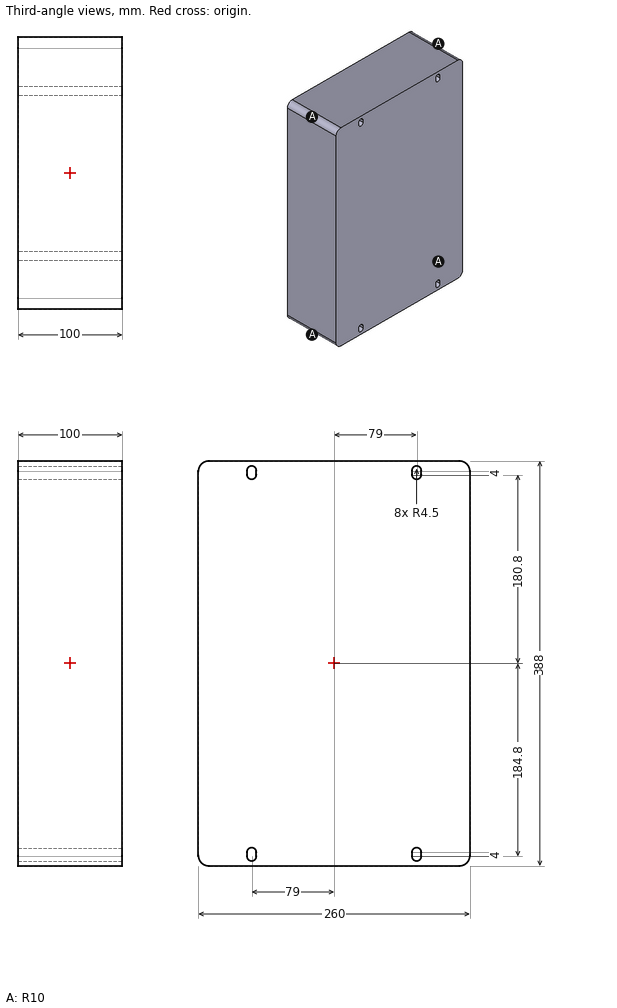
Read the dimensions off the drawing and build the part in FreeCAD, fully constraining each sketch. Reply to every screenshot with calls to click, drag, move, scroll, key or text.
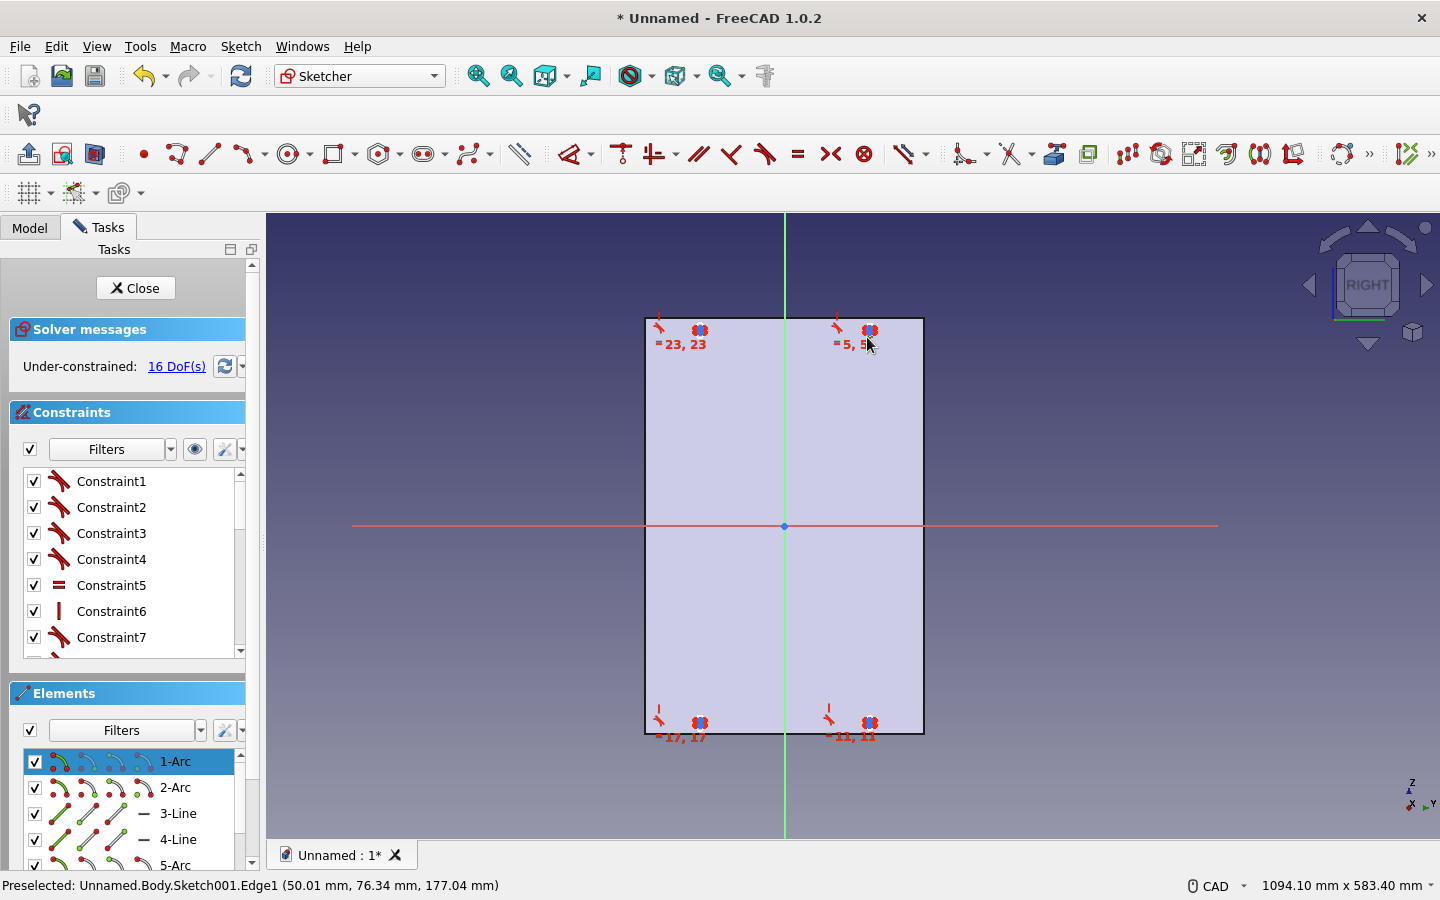
scroll(867, 729, up, 6)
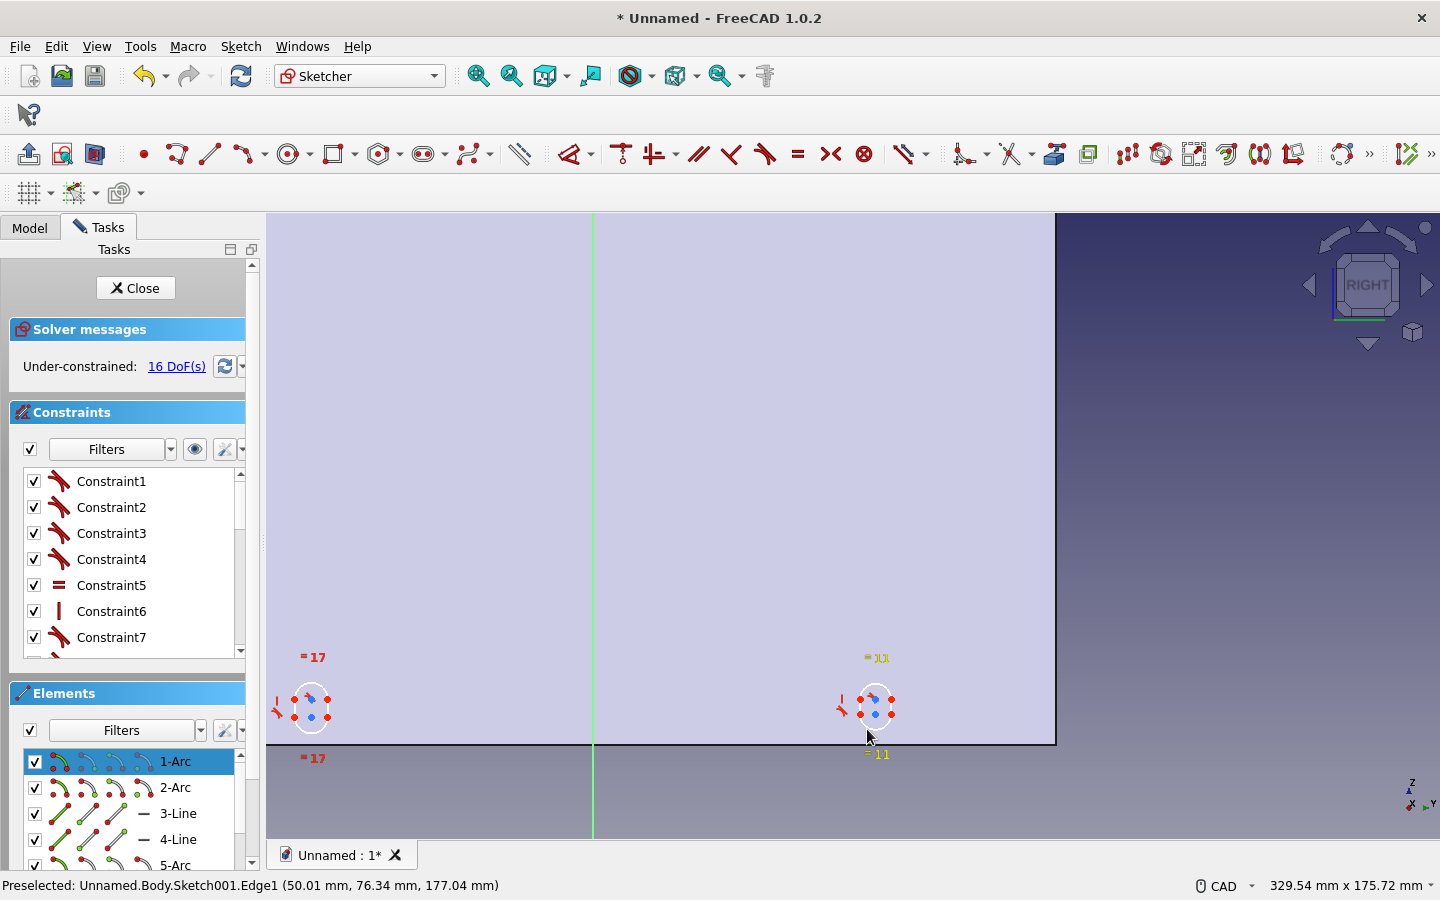
click(866, 727)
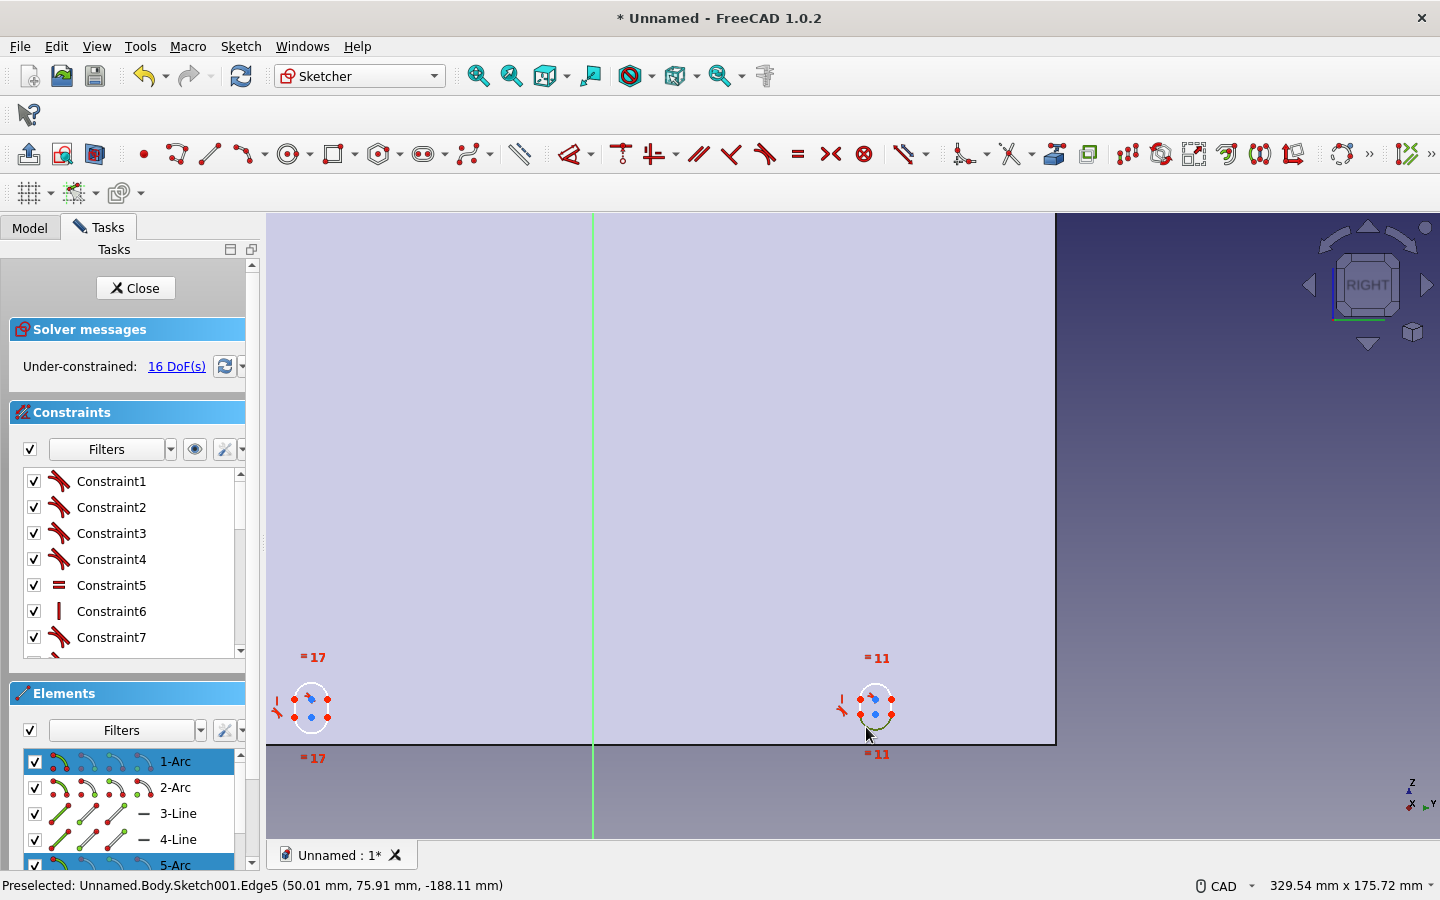
click(302, 730)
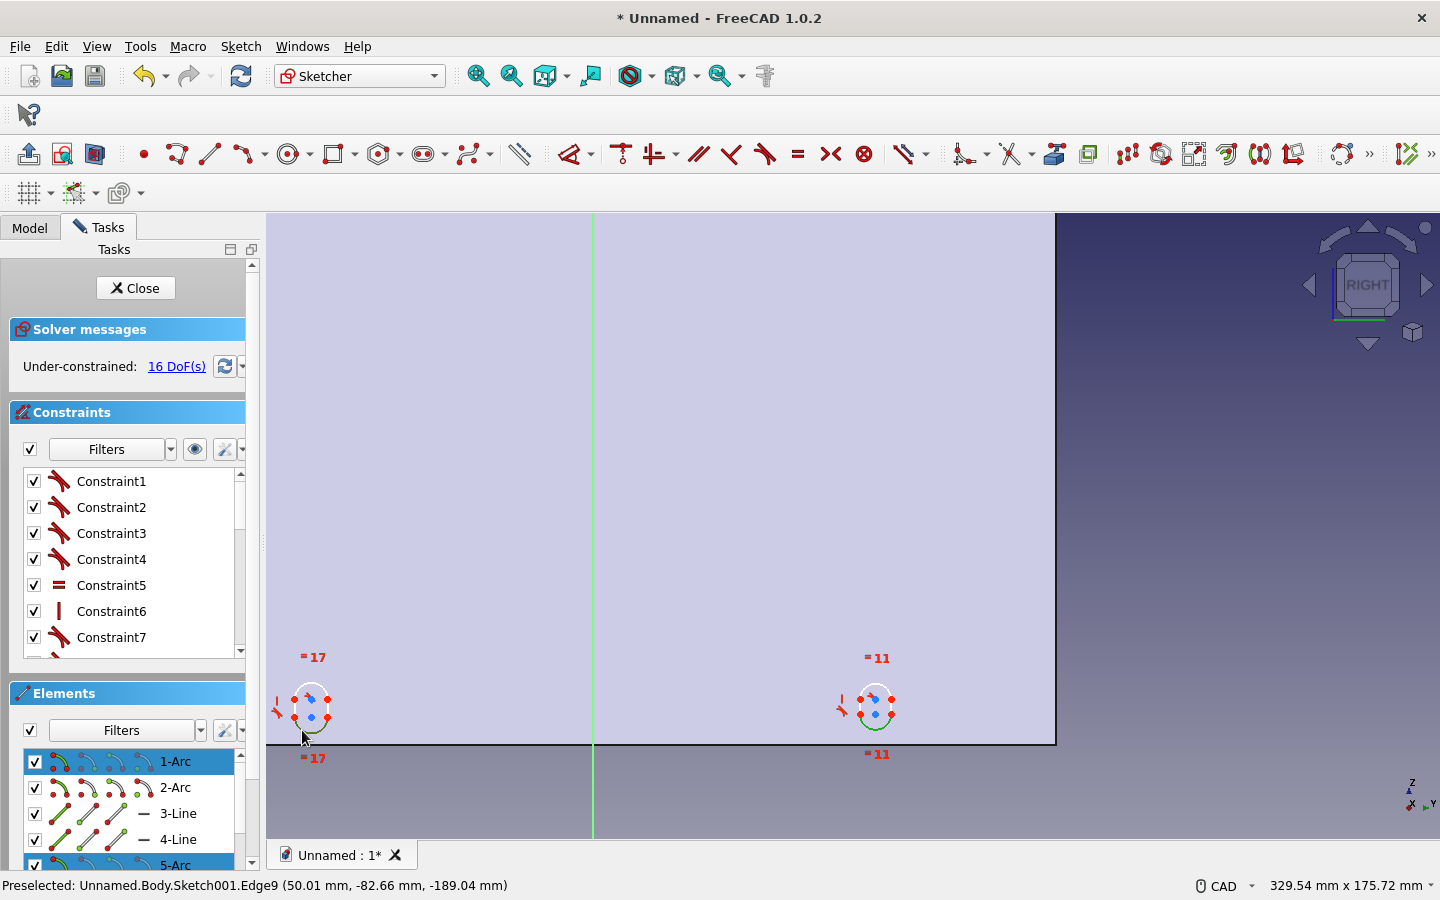
scroll(867, 729, down, 6)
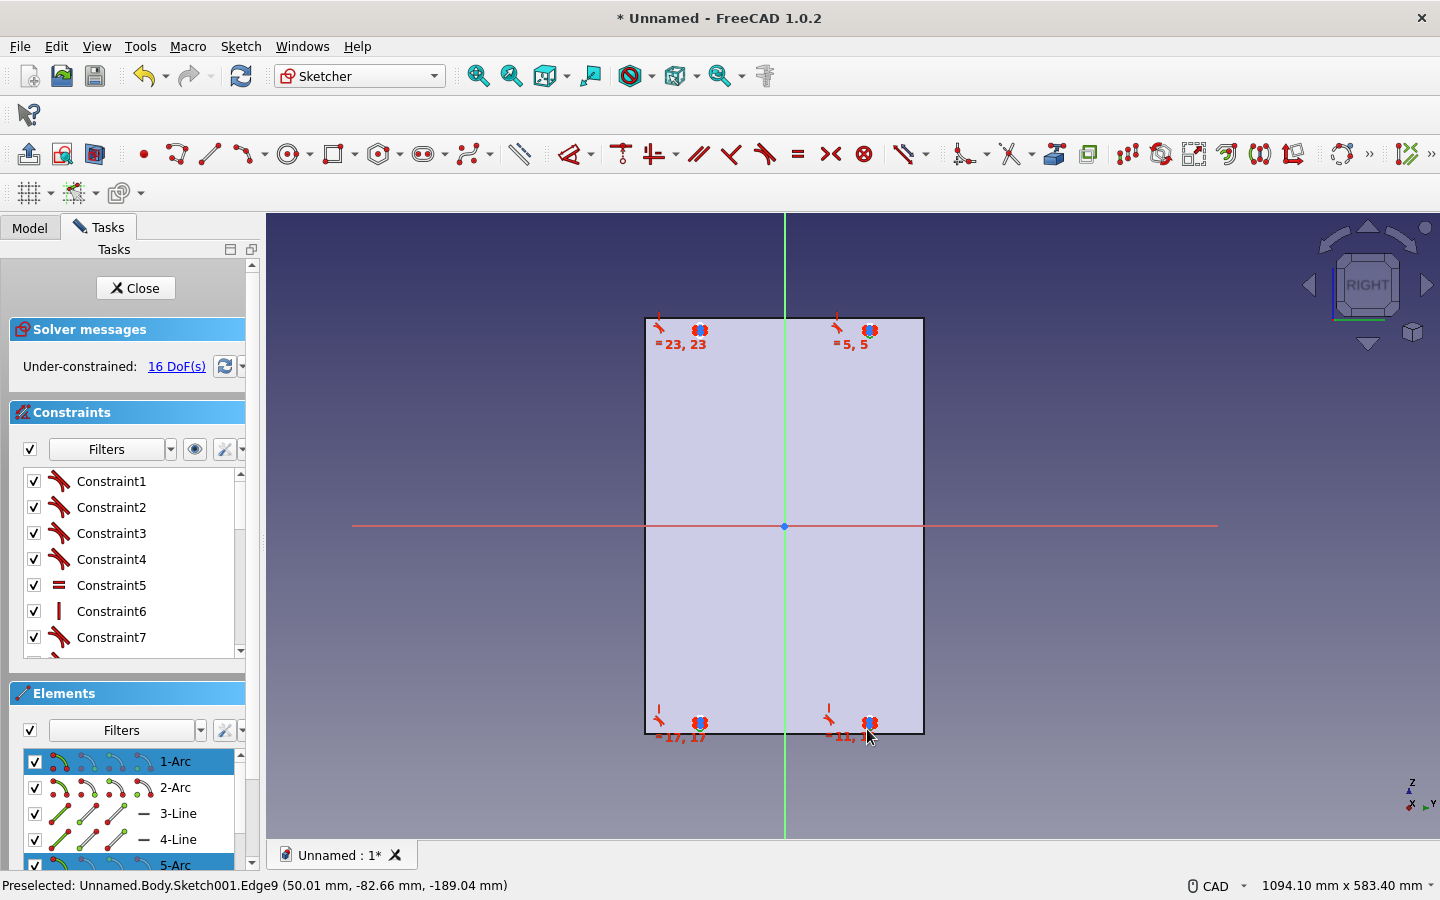
scroll(697, 337, up, 6)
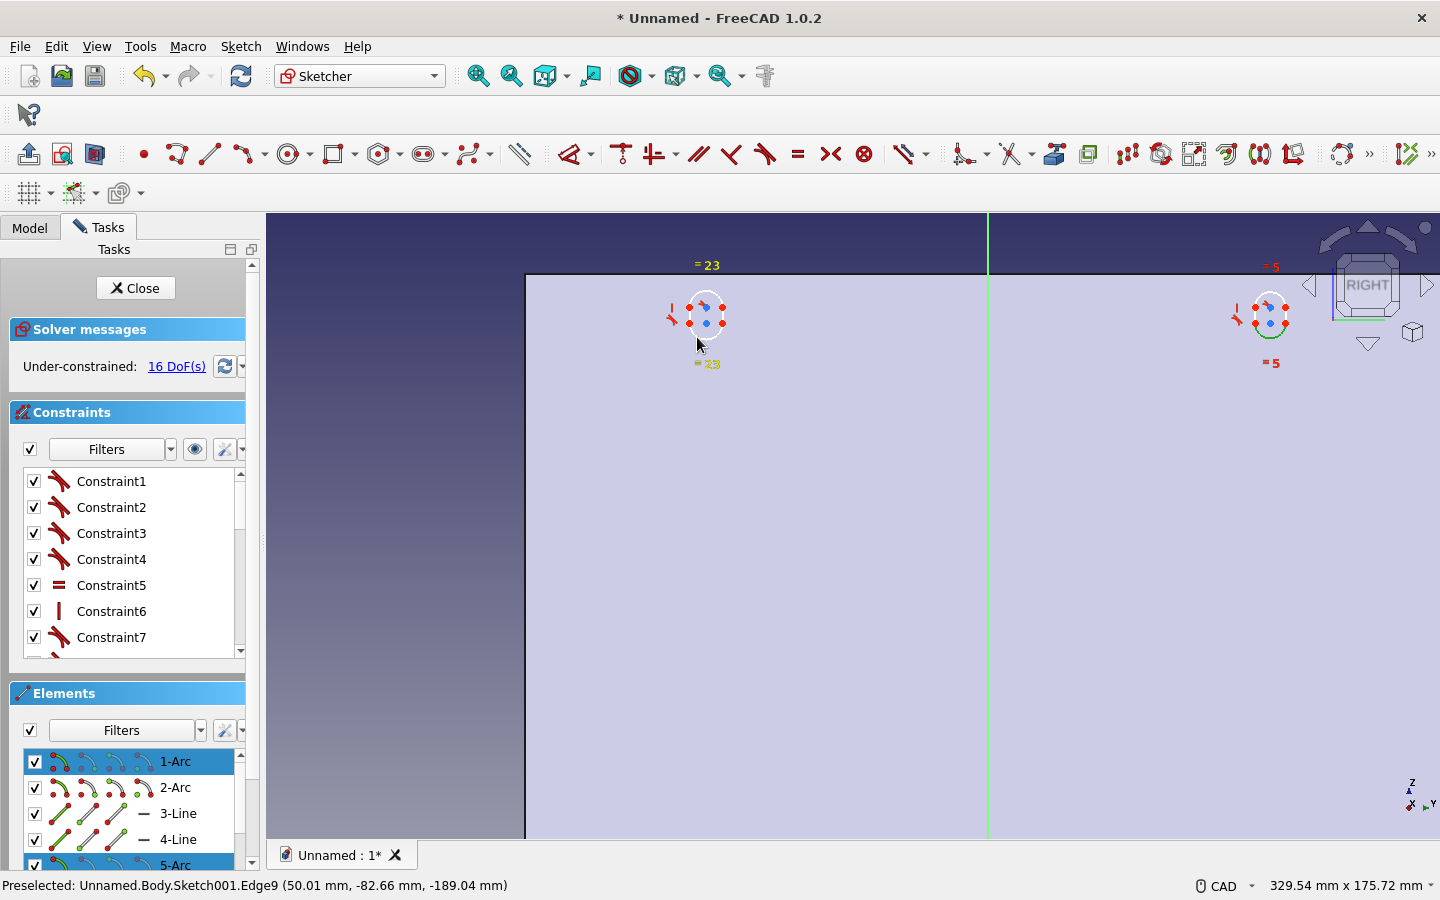
click(697, 336)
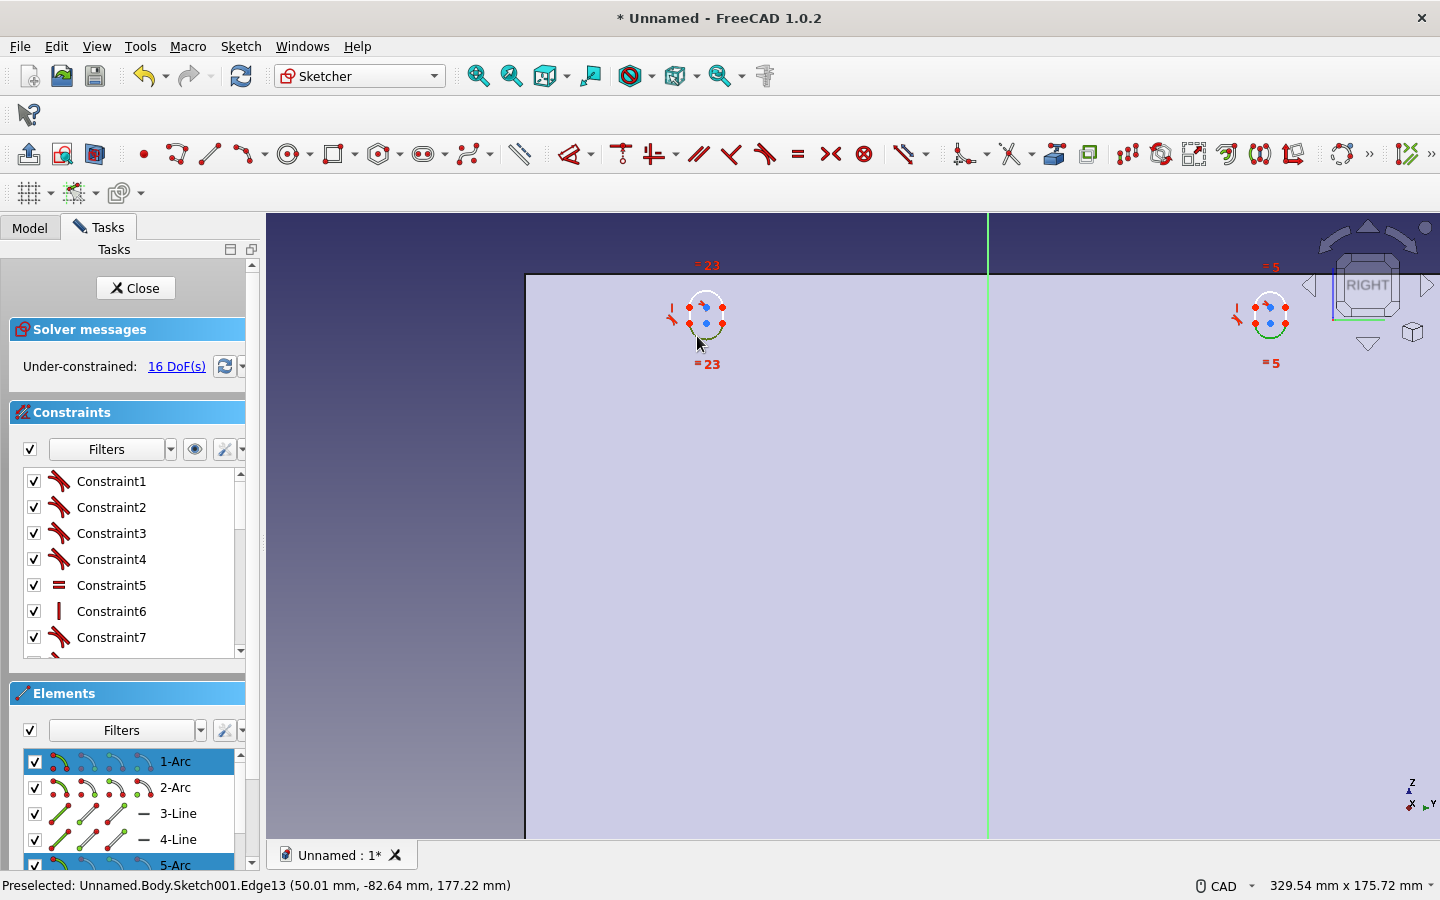
key(e)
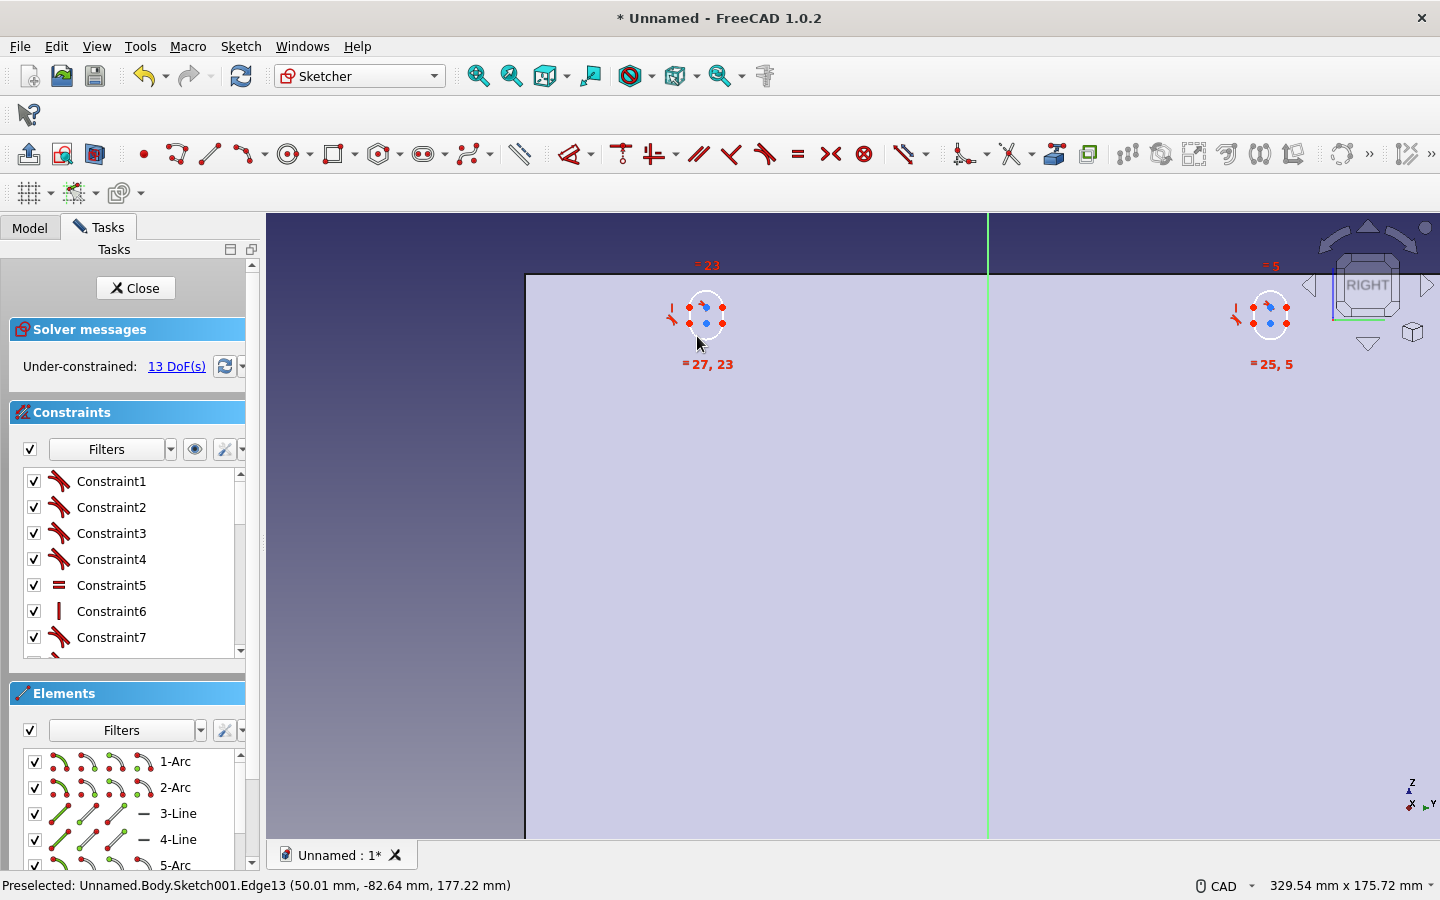
key(d)